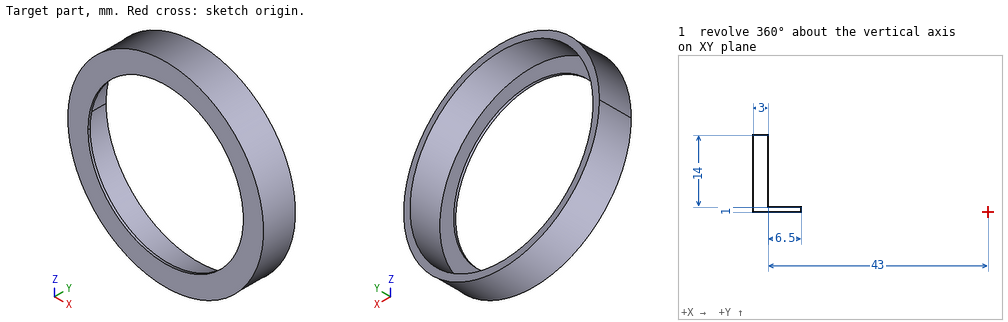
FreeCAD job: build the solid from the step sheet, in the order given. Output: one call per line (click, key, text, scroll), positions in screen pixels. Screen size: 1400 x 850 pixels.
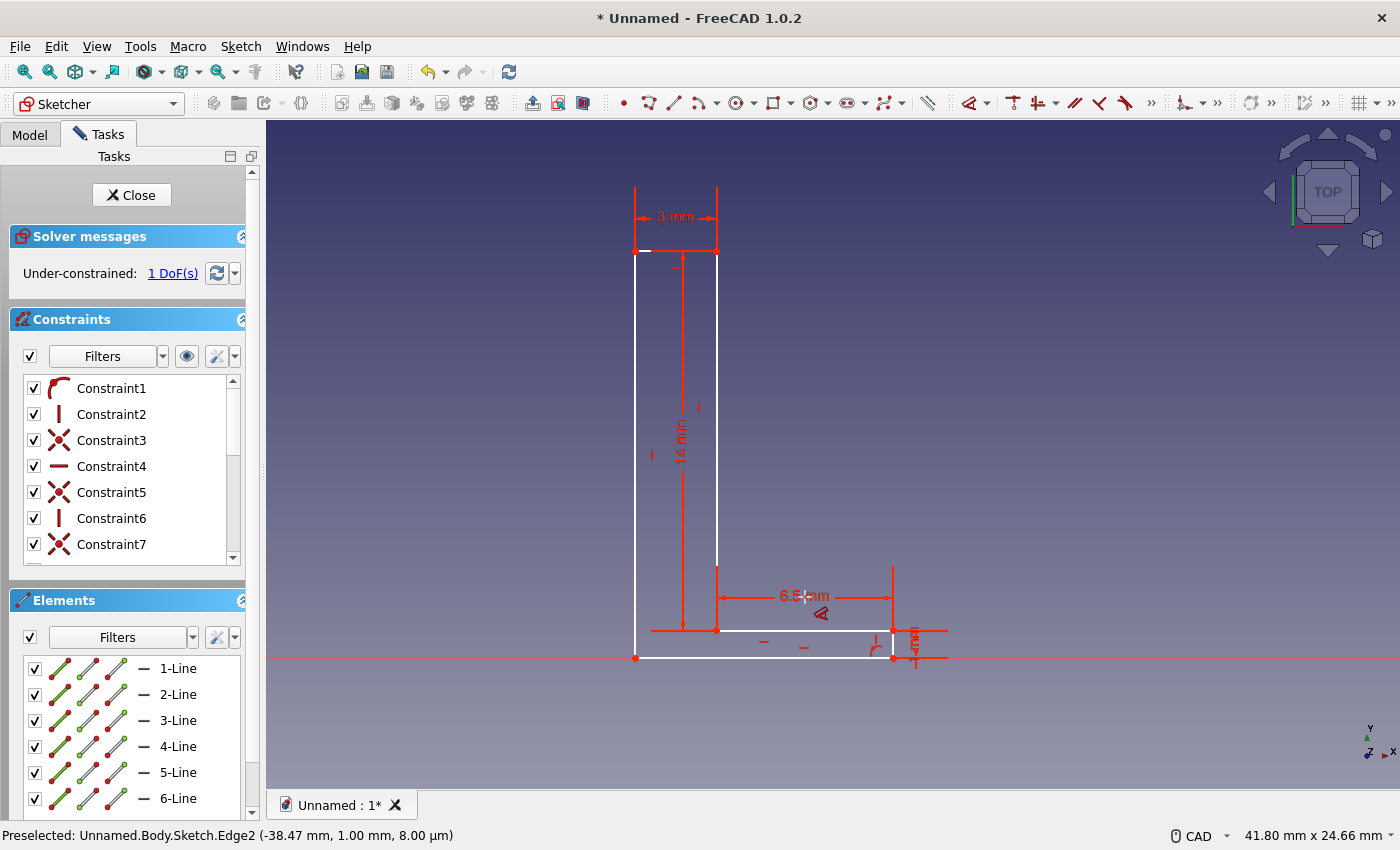
click(717, 631)
click(976, 692)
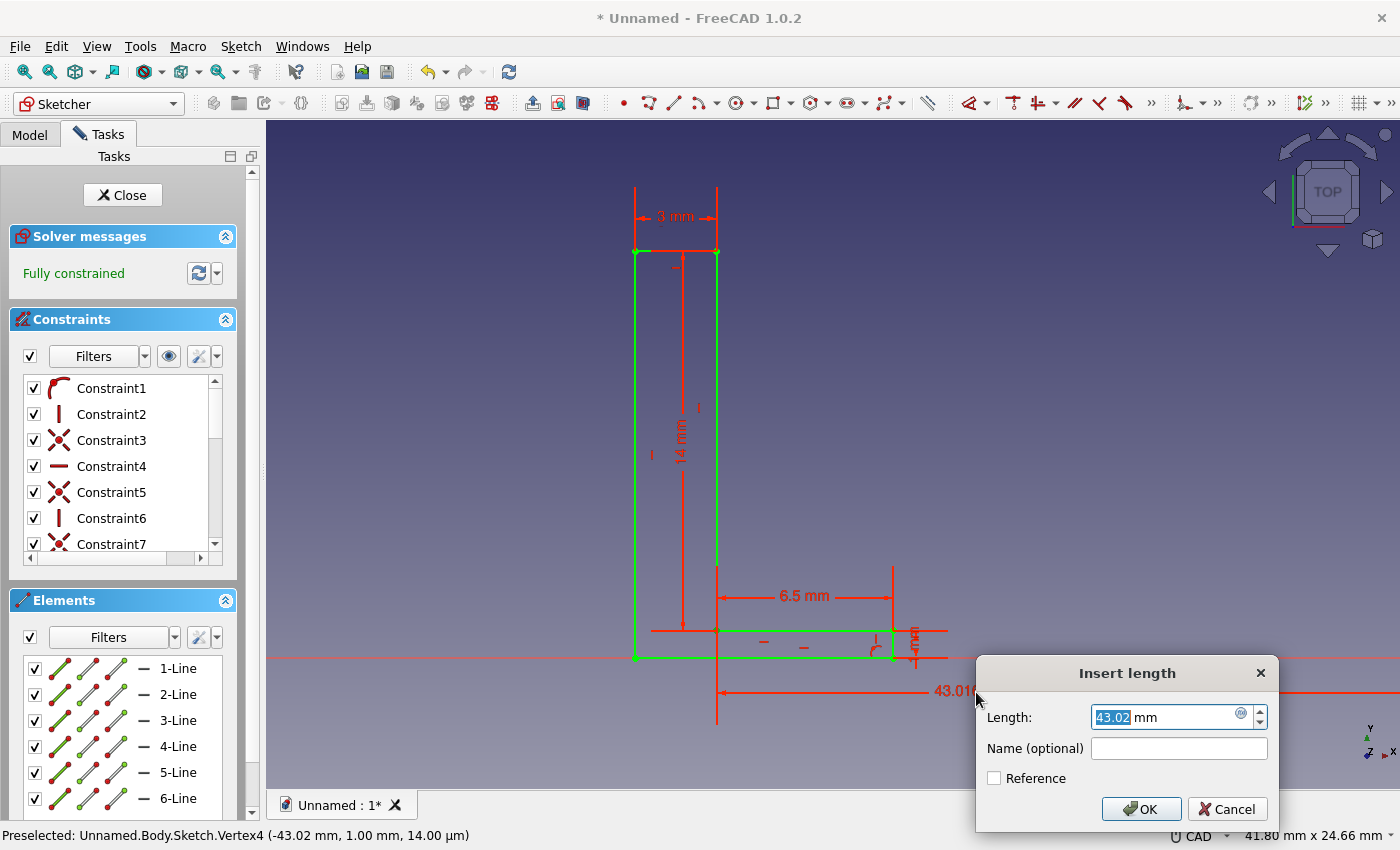
text(43)
key(Return)
key(Escape)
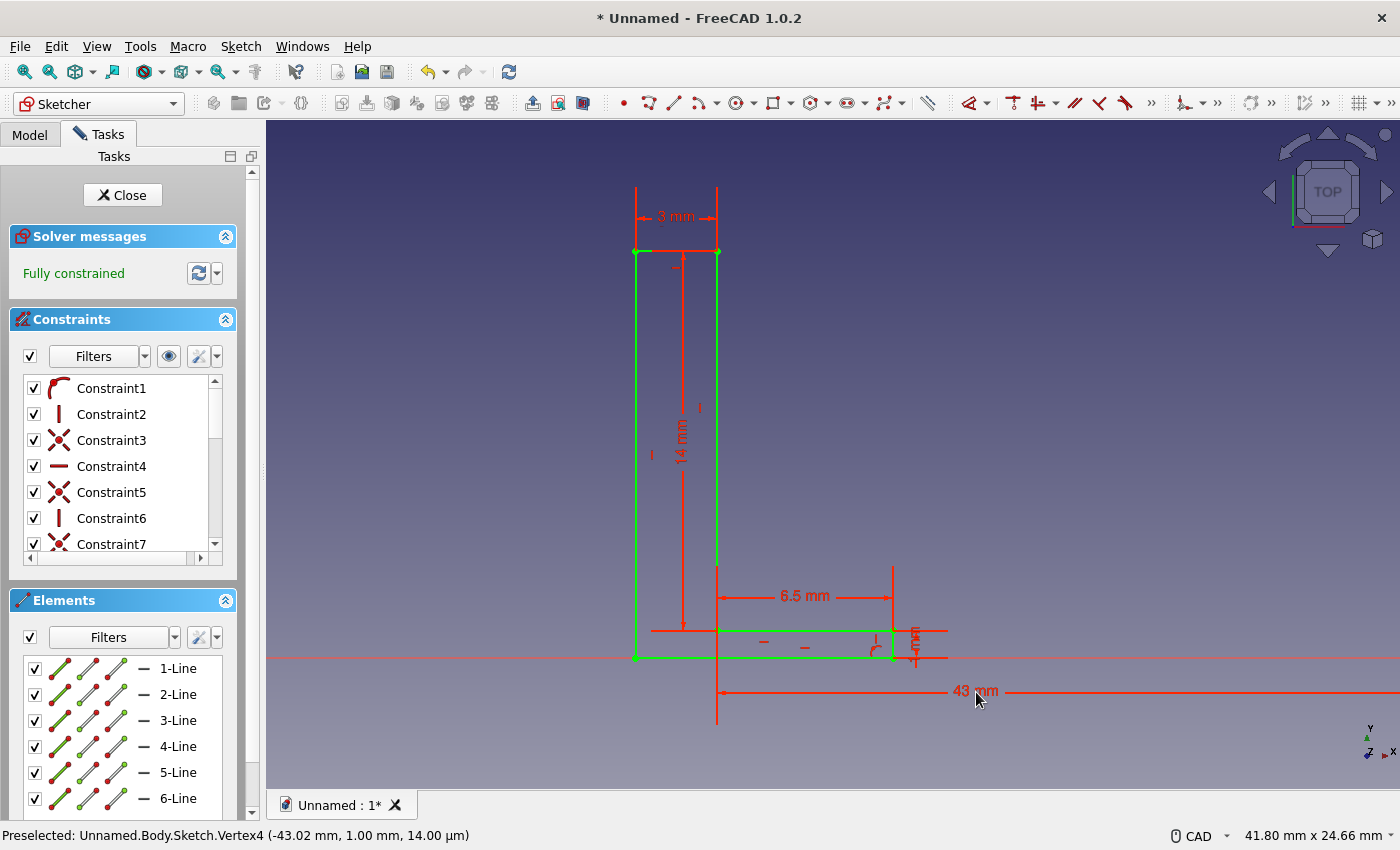
click(123, 195)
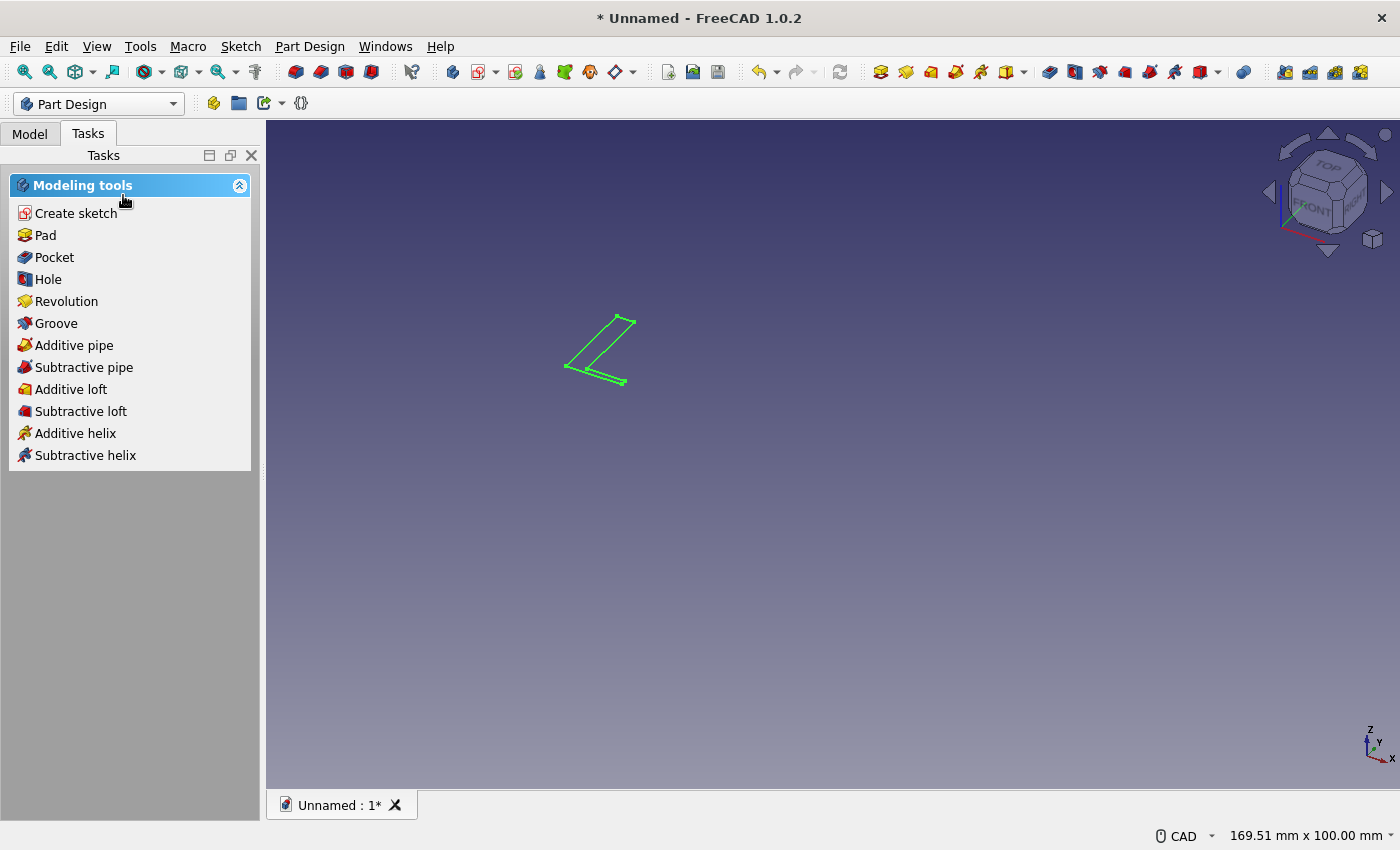
click(906, 72)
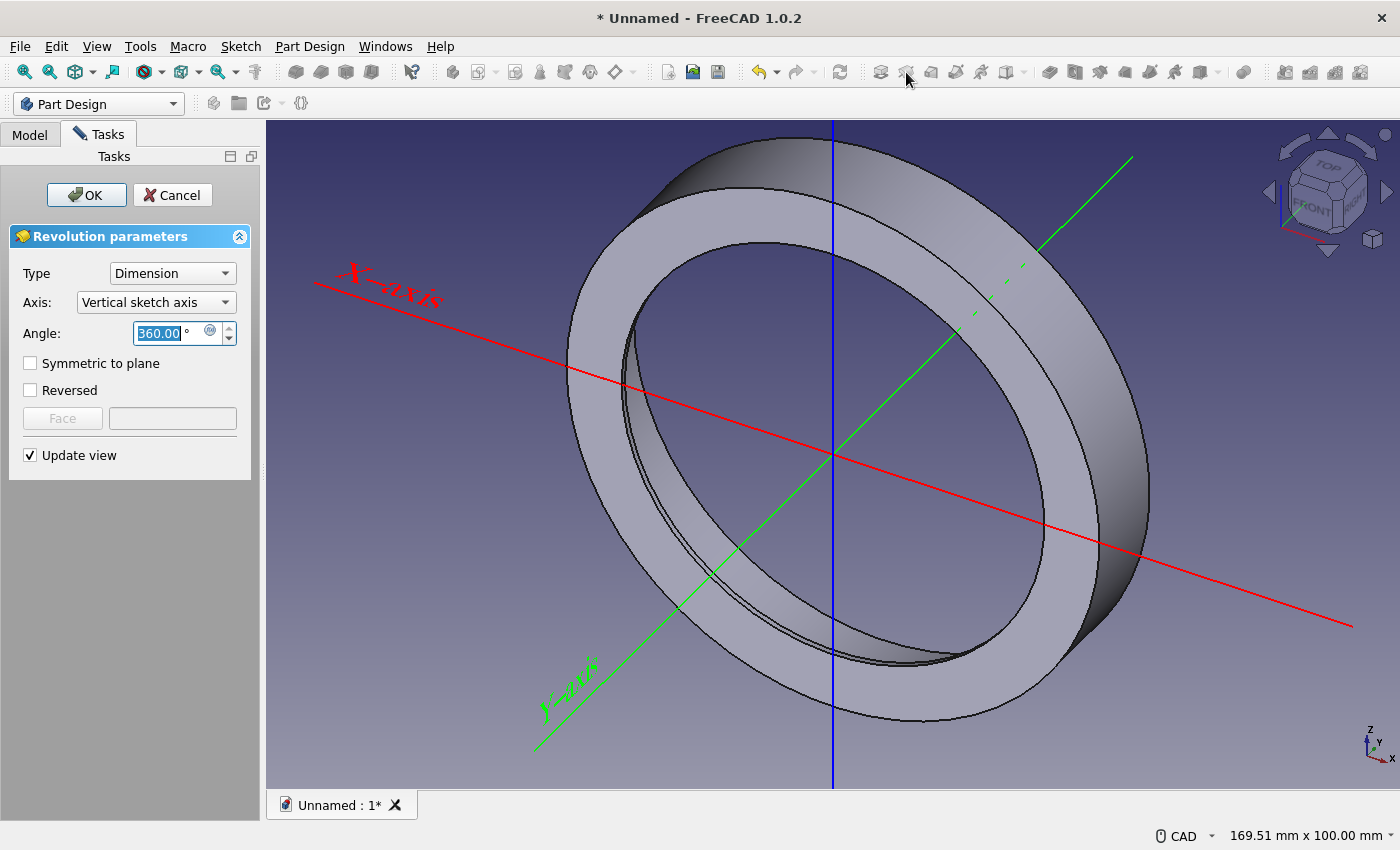
click(87, 195)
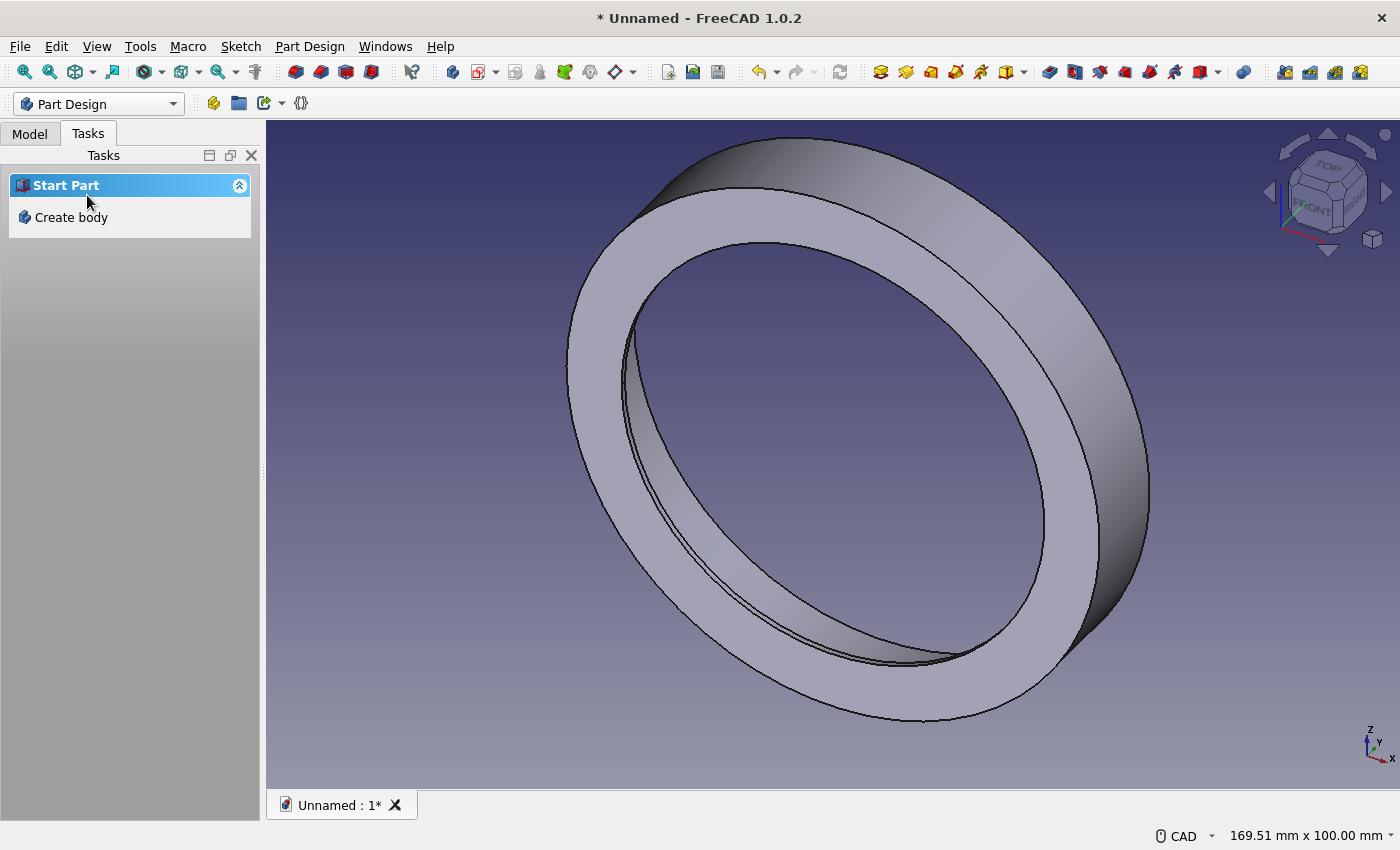
key(0)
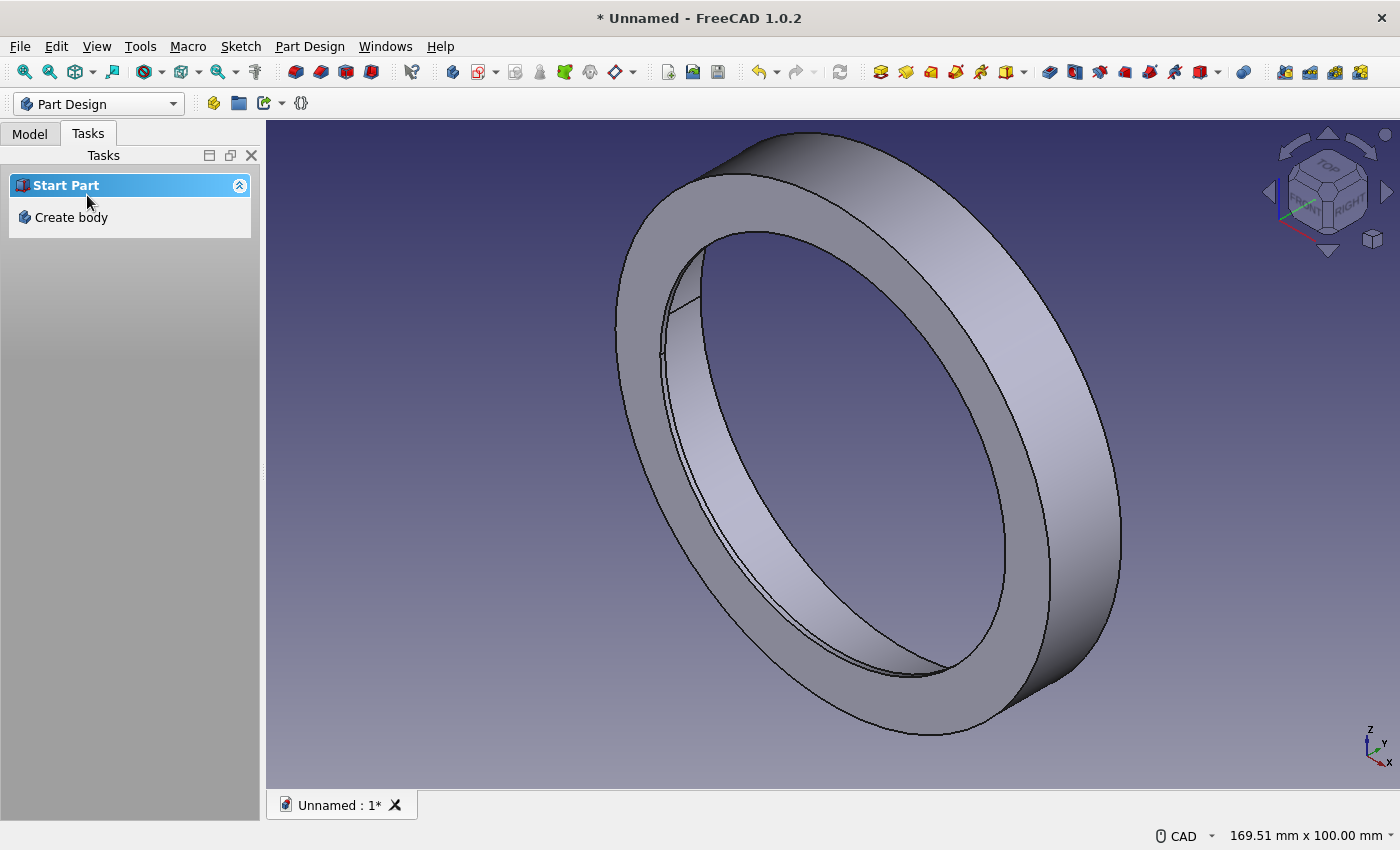
click(25, 72)